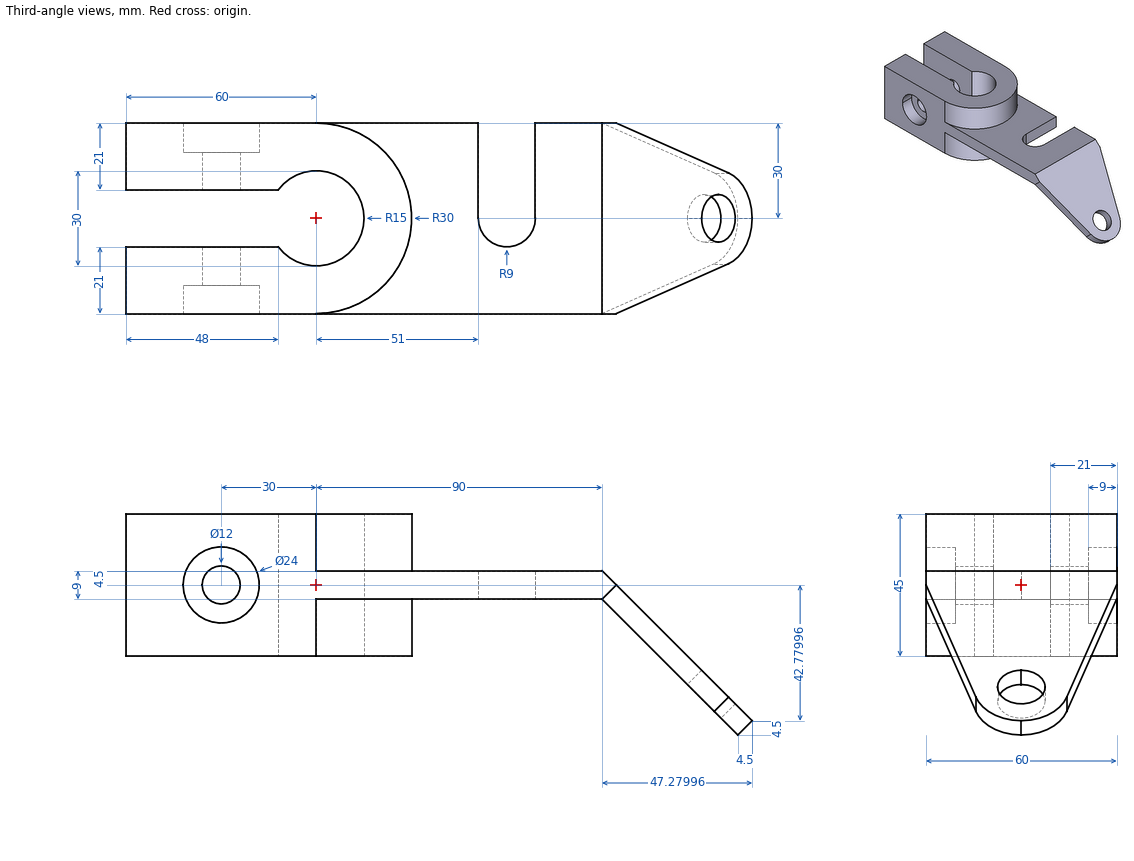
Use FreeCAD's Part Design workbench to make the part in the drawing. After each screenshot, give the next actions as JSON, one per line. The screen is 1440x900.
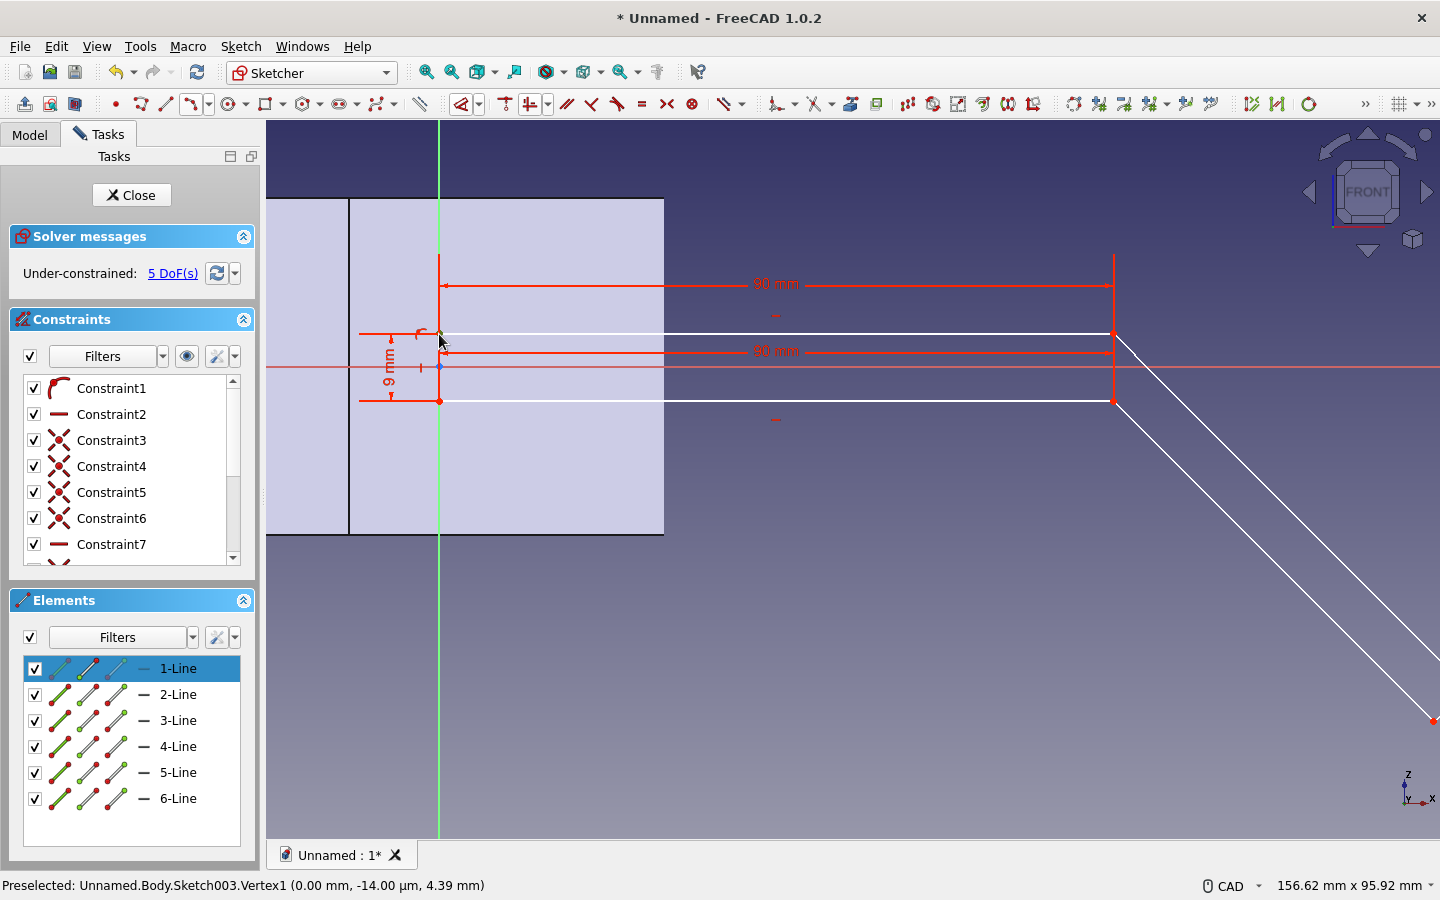
{"action": "left_click", "coordinate": [478, 104]}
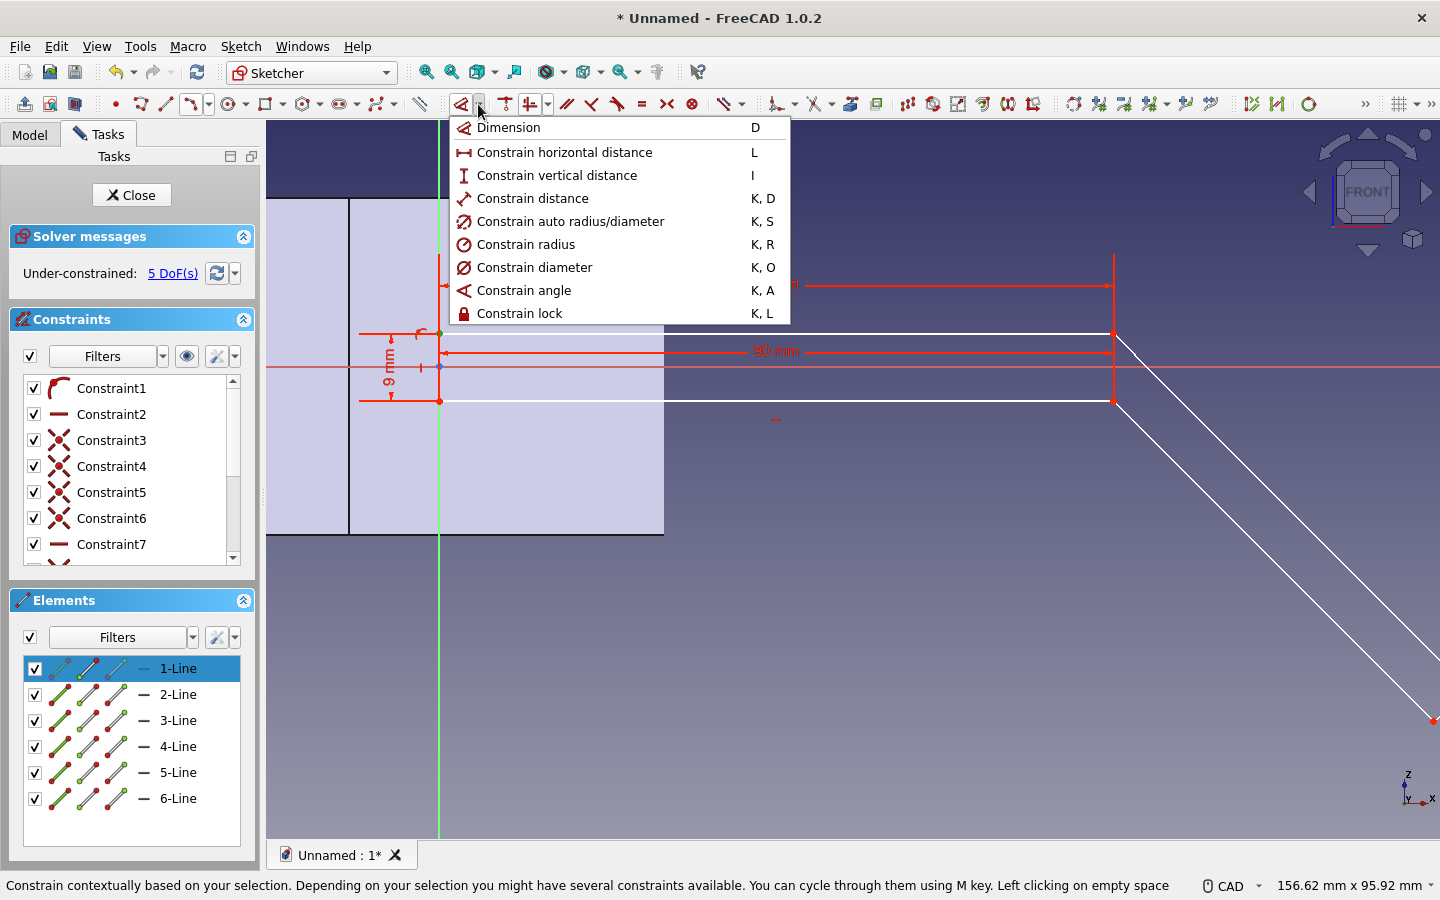
{"action": "left_click", "coordinate": [620, 176]}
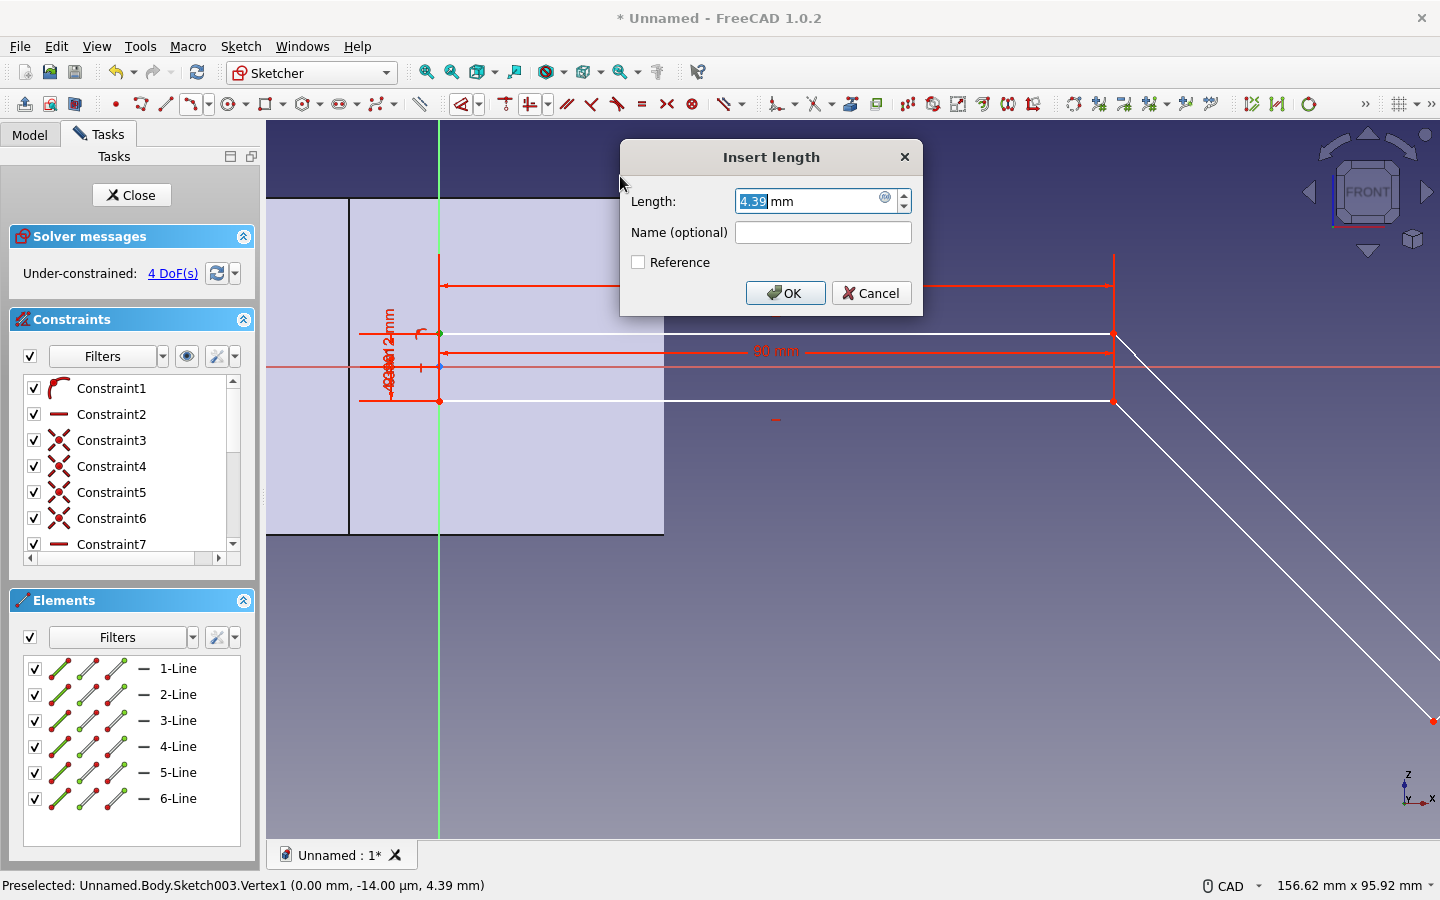
{"action": "type", "text": "4.5"}
{"action": "key", "text": "Return"}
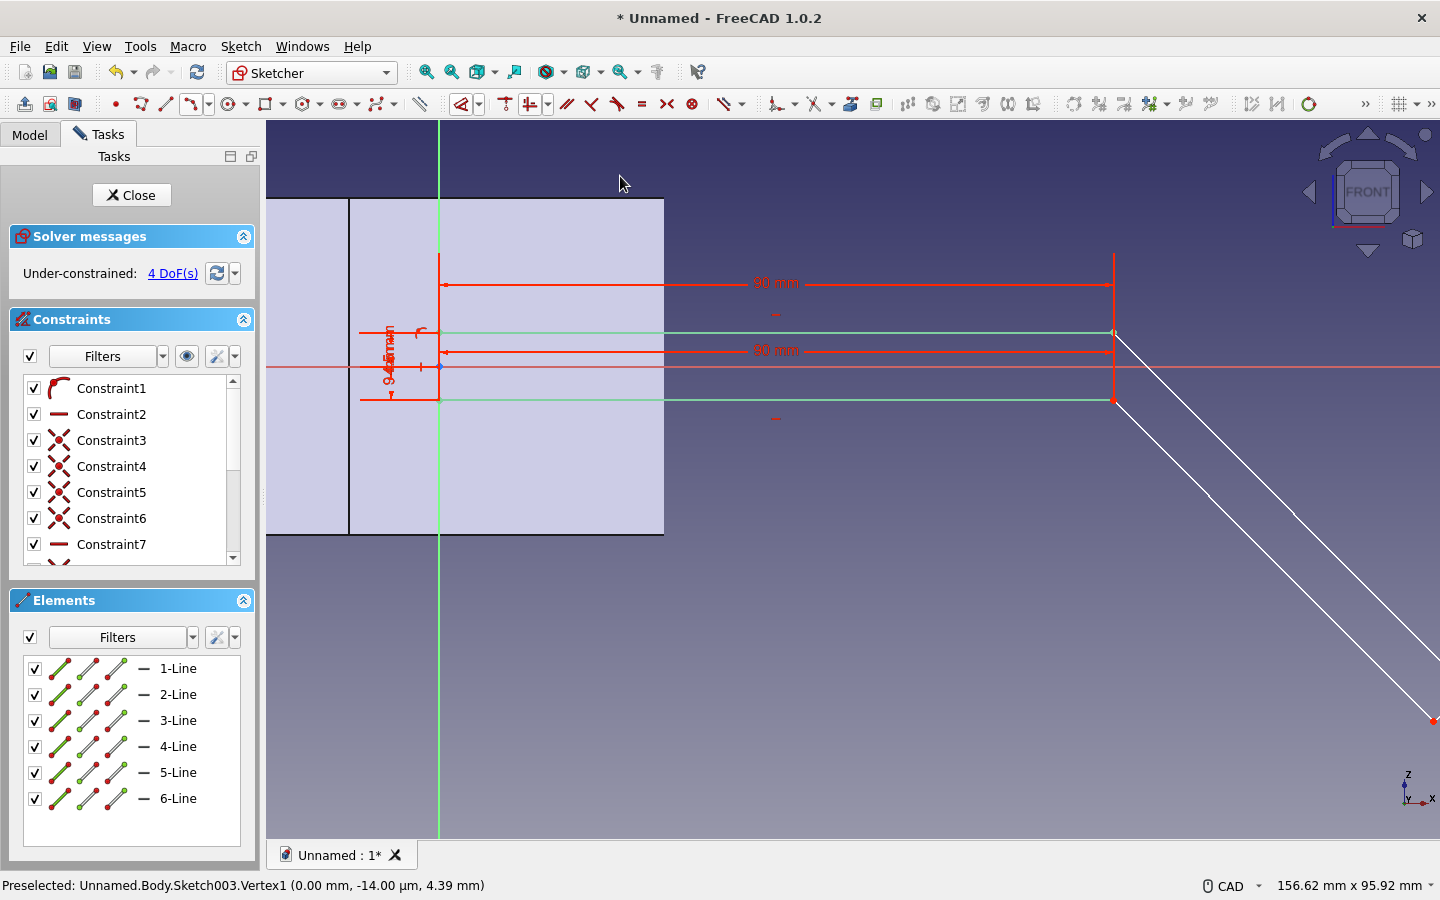
{"action": "scroll", "coordinate": [440, 383], "scroll_direction": "down", "scroll_amount": 2}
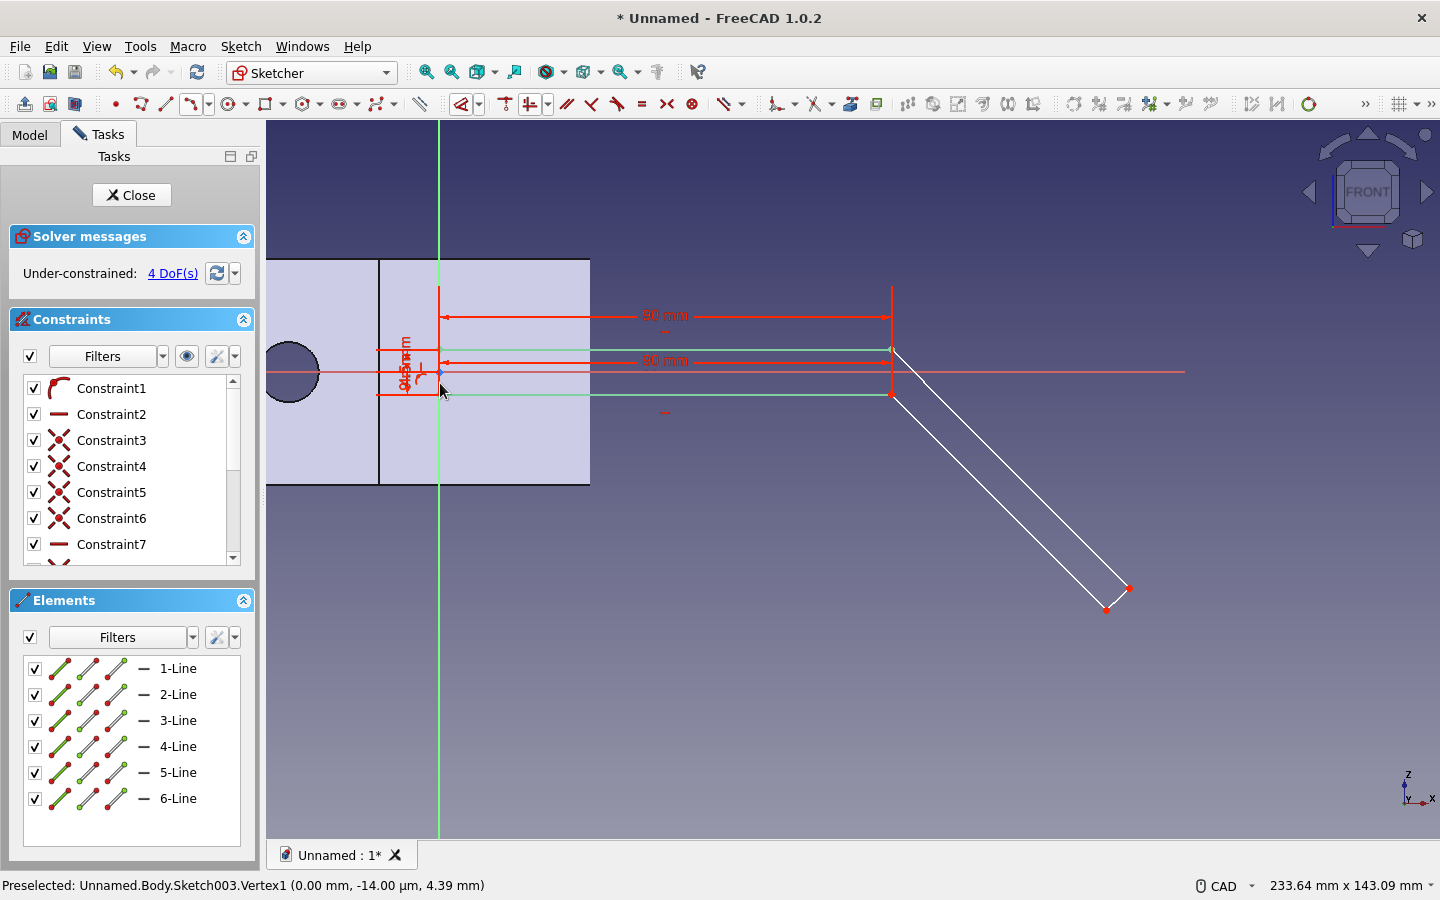
{"action": "scroll", "coordinate": [1122, 595], "scroll_direction": "up", "scroll_amount": 3}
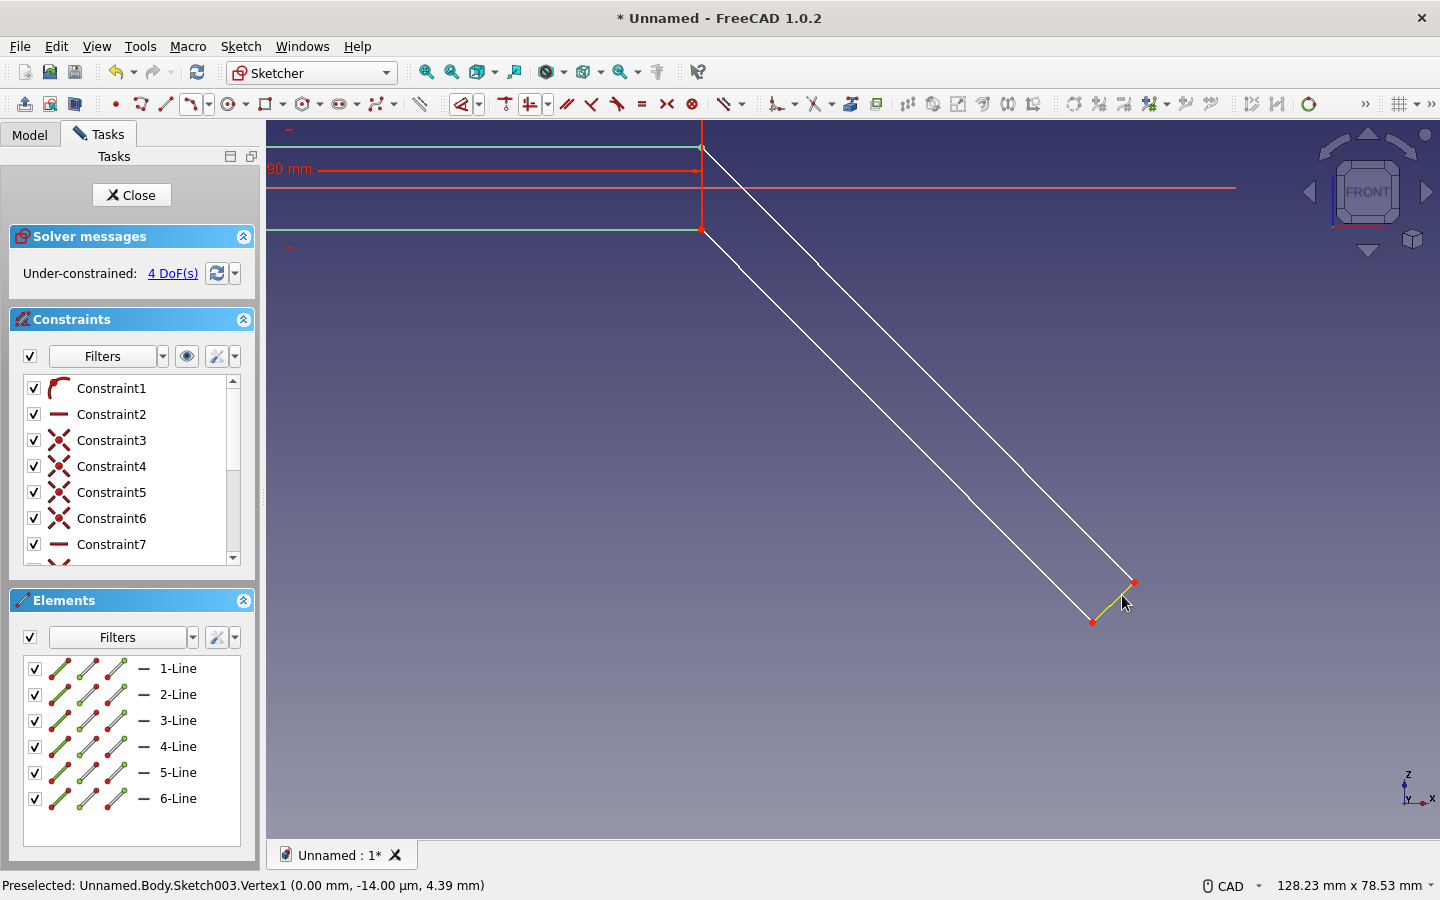
{"action": "left_click", "coordinate": [1122, 594]}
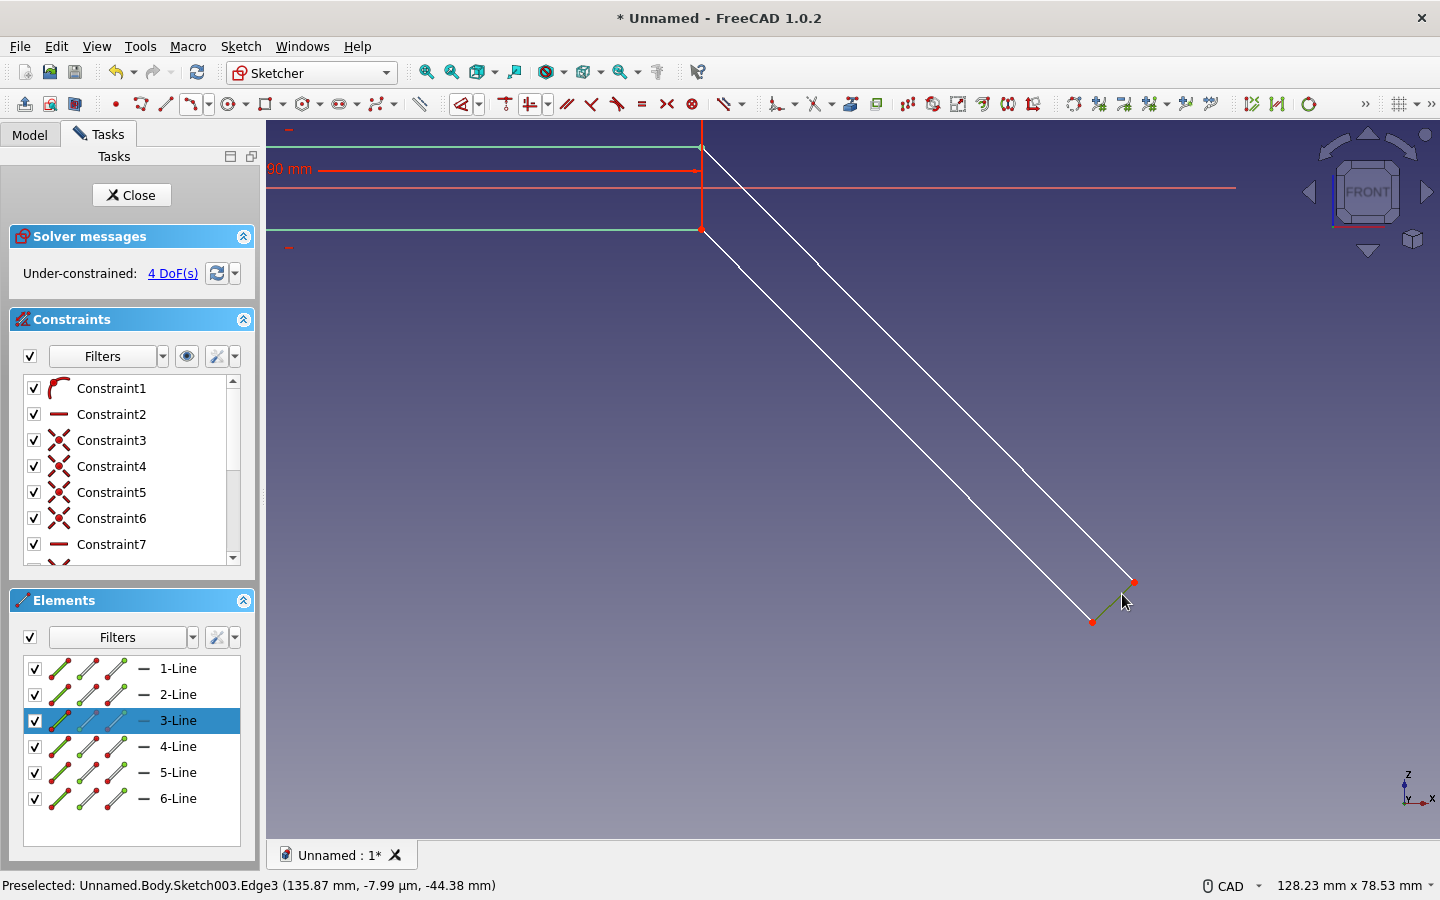
{"action": "key", "text": "l"}